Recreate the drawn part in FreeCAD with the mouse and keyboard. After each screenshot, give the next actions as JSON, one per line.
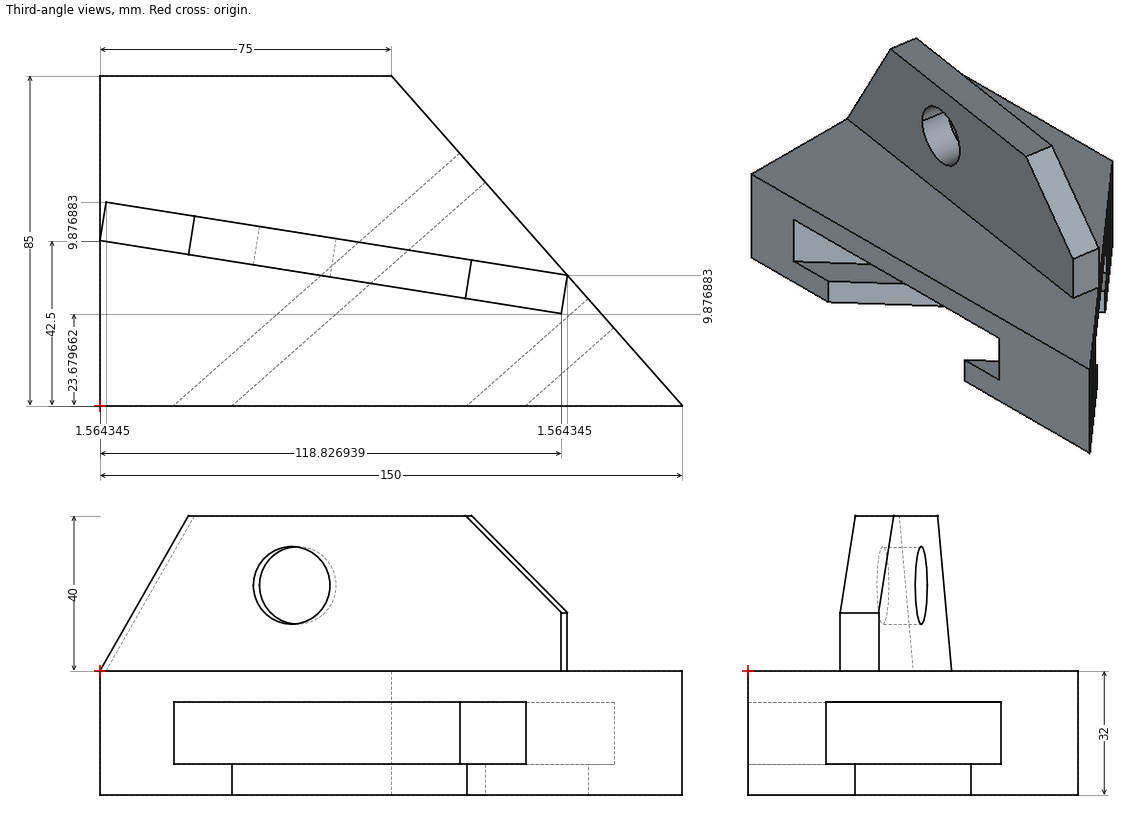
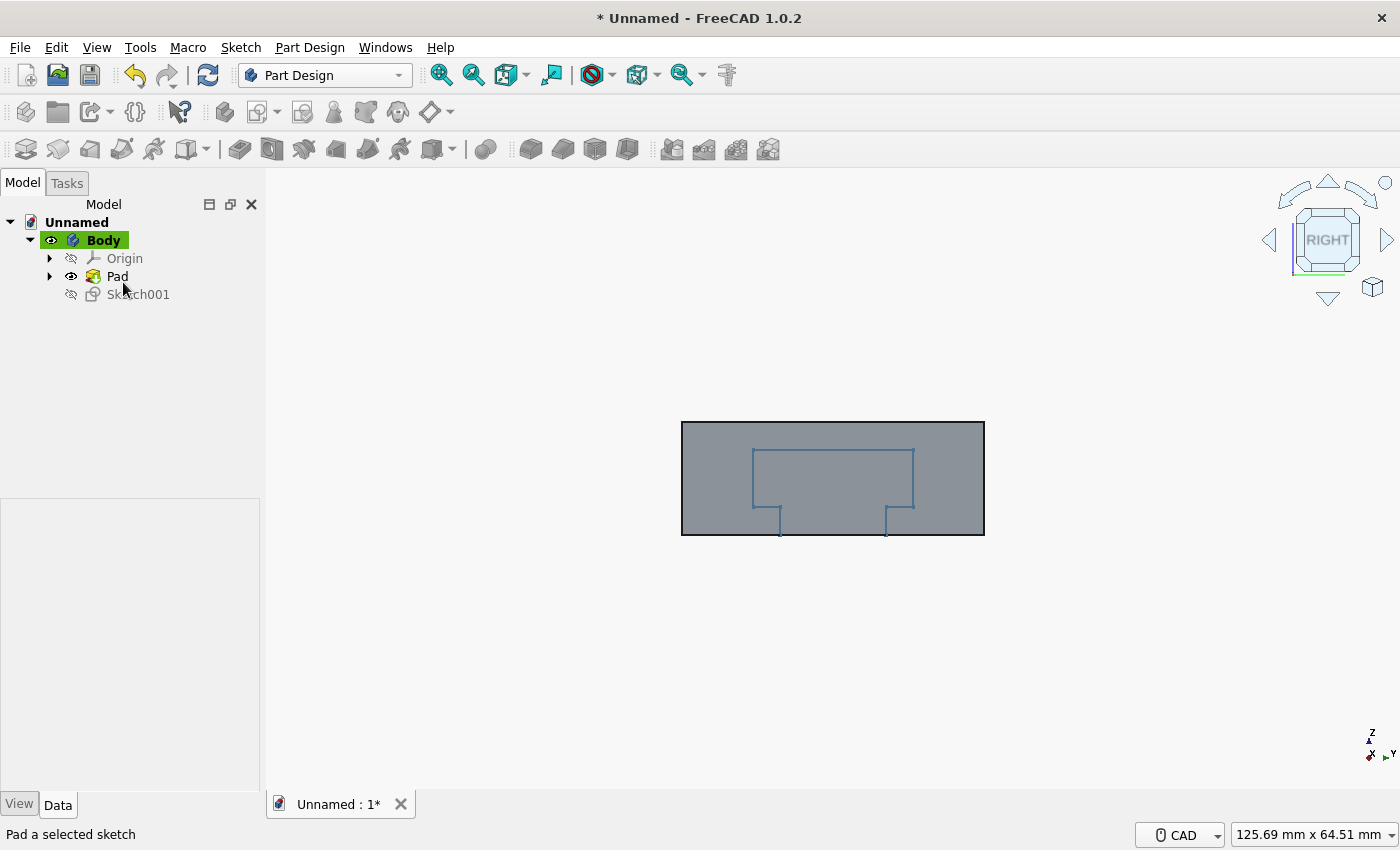
{"action": "left_click", "coordinate": [240, 150]}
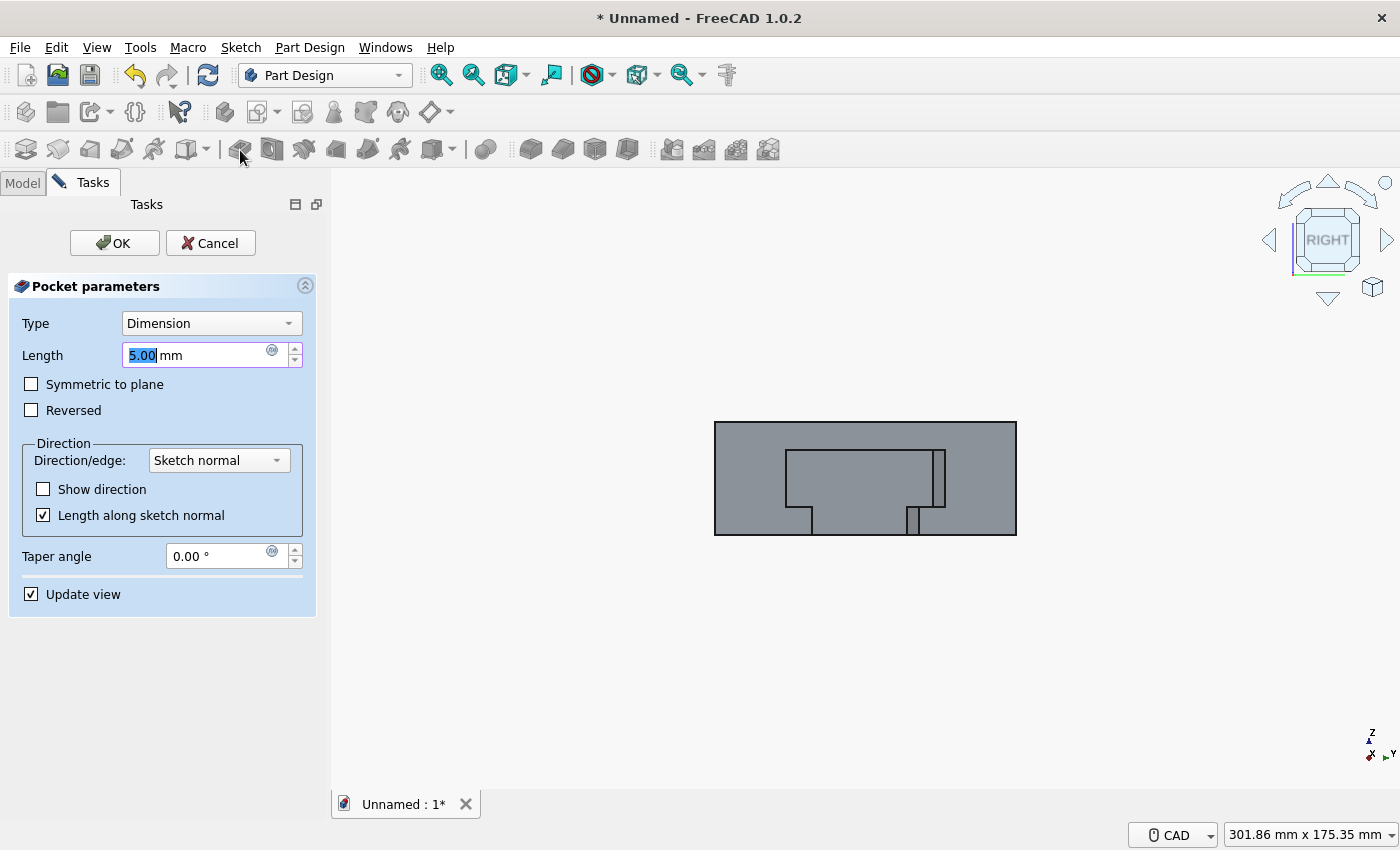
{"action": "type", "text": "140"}
{"action": "key", "text": "Tab"}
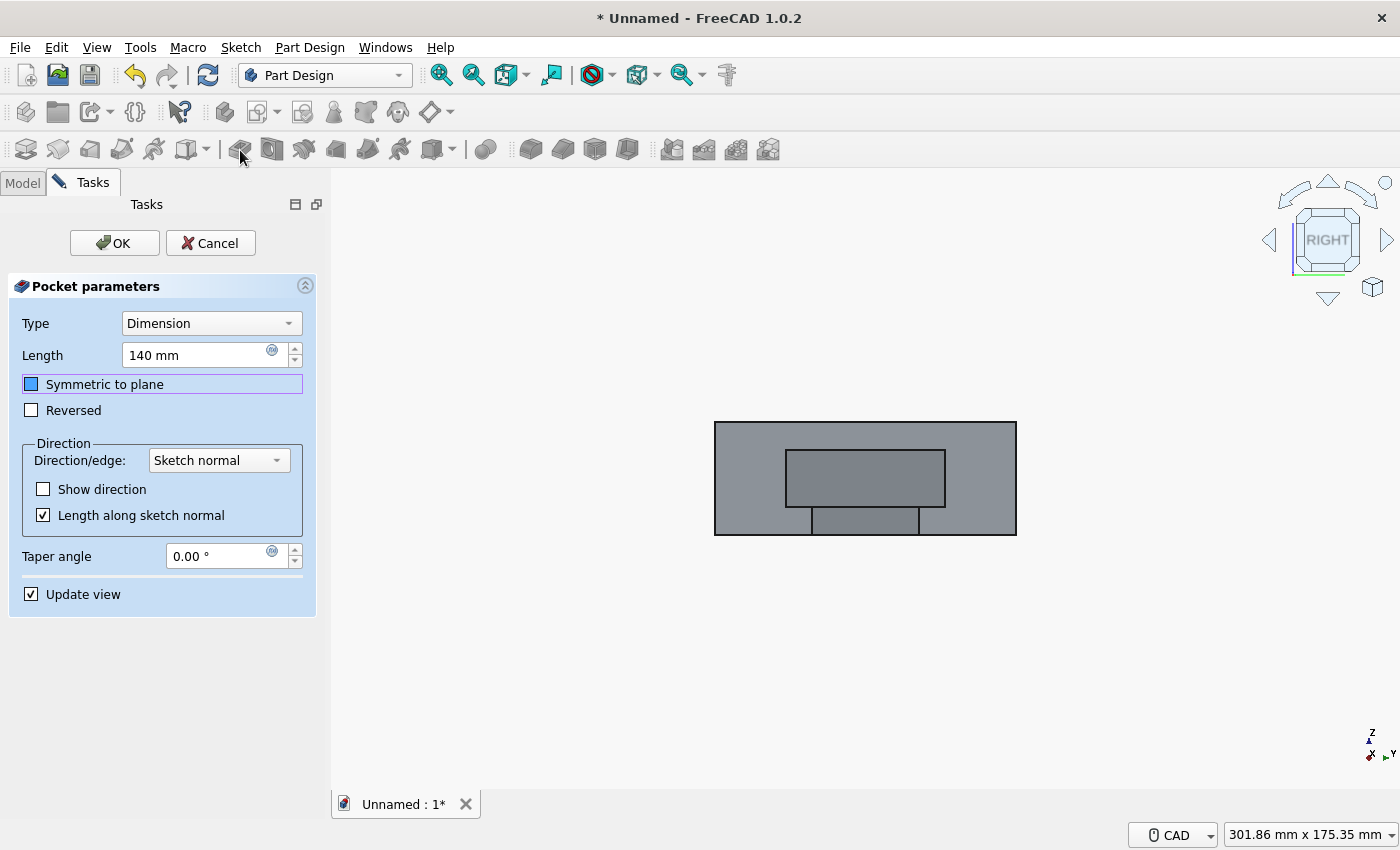
{"action": "left_click", "coordinate": [115, 243]}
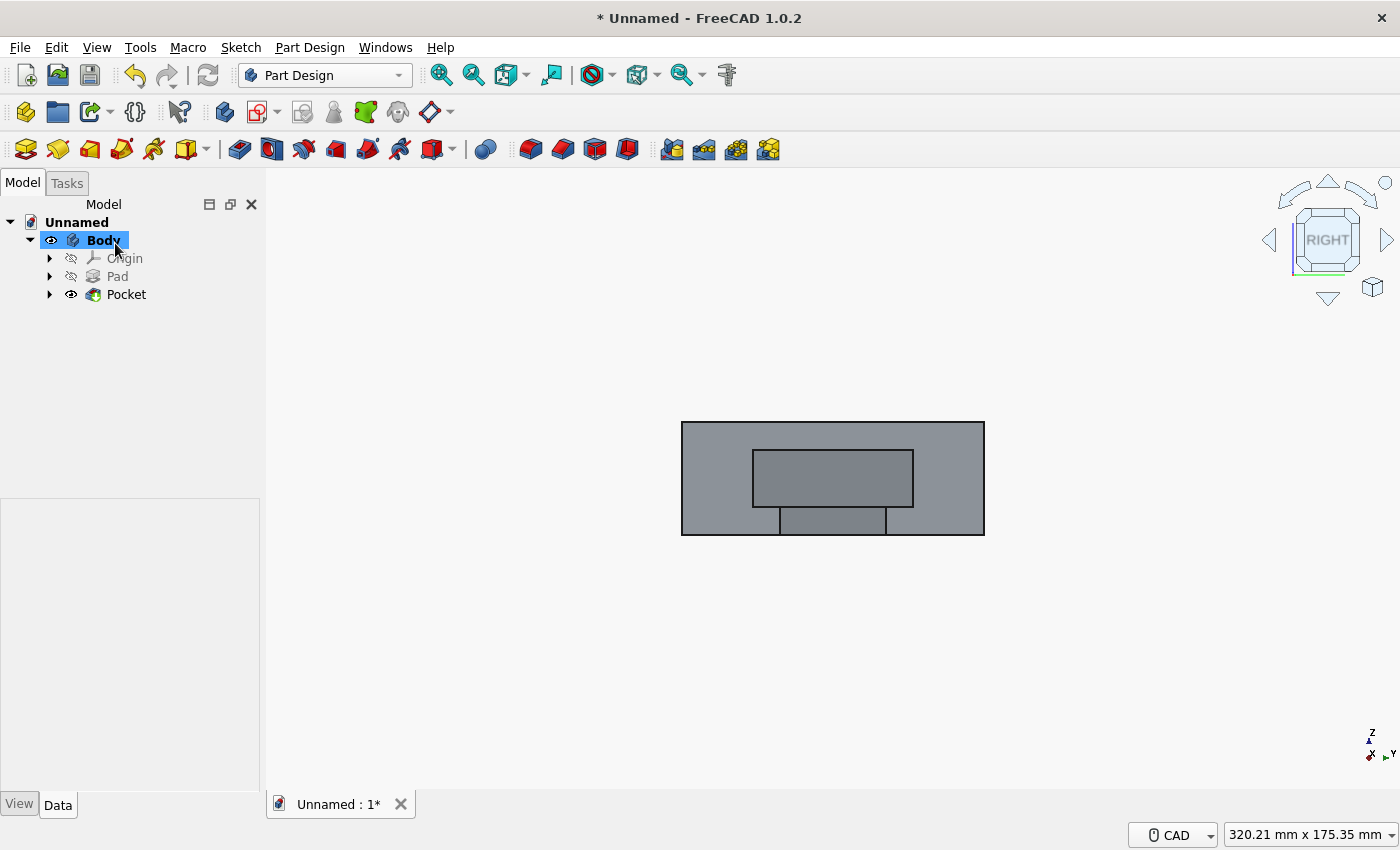
{"action": "key", "text": "v f"}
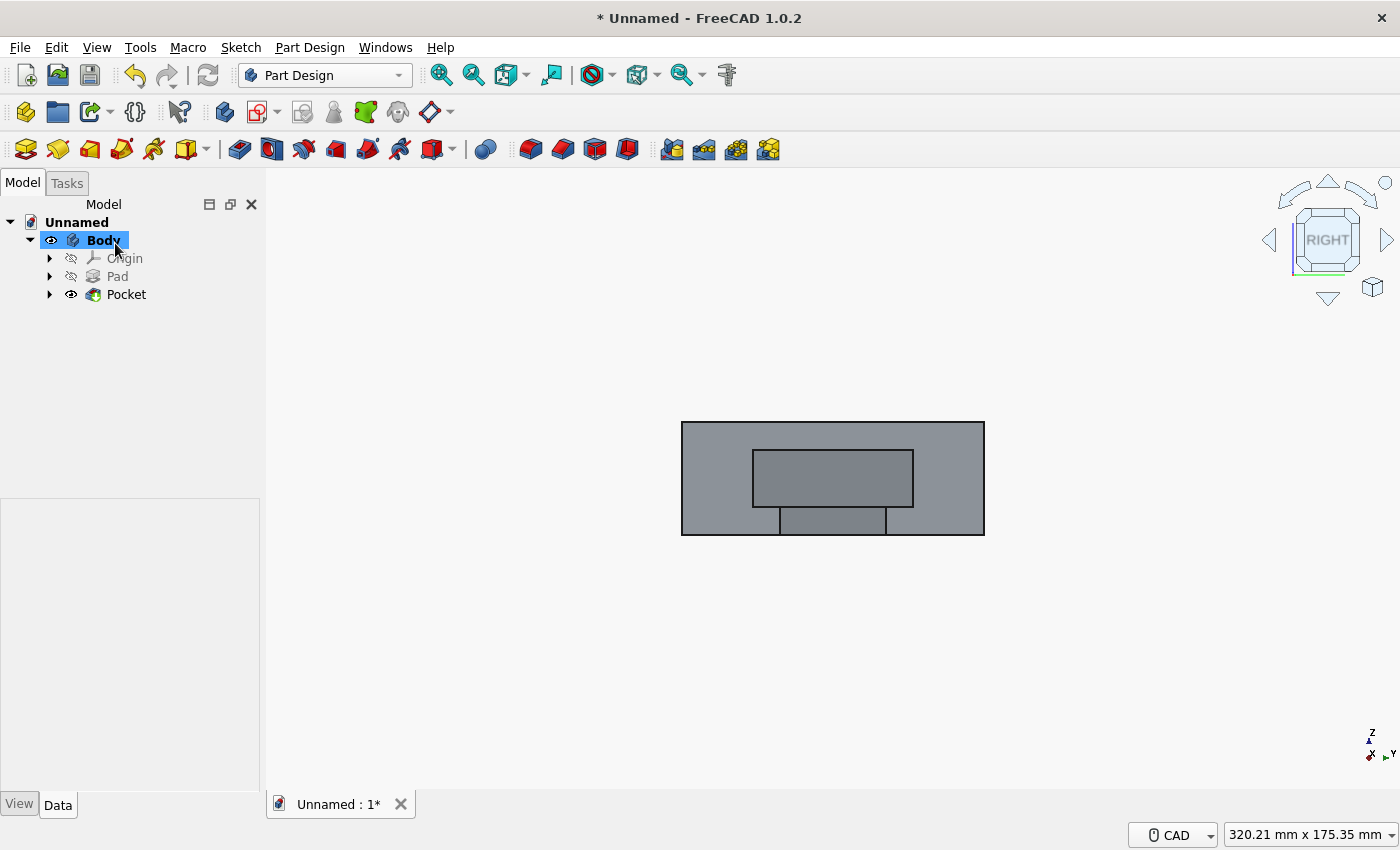
{"action": "key", "text": "0"}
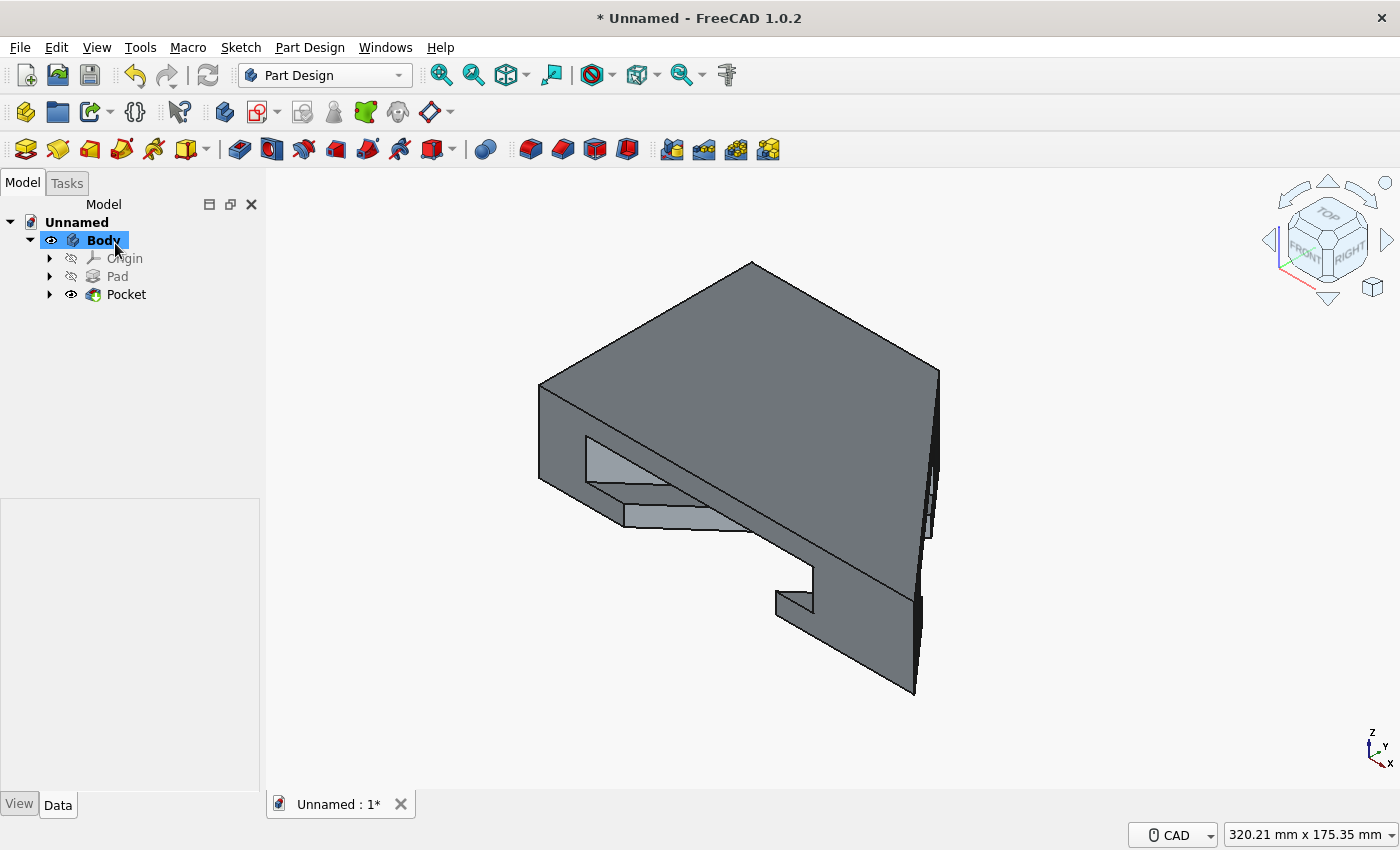
{"action": "left_click", "coordinate": [779, 400]}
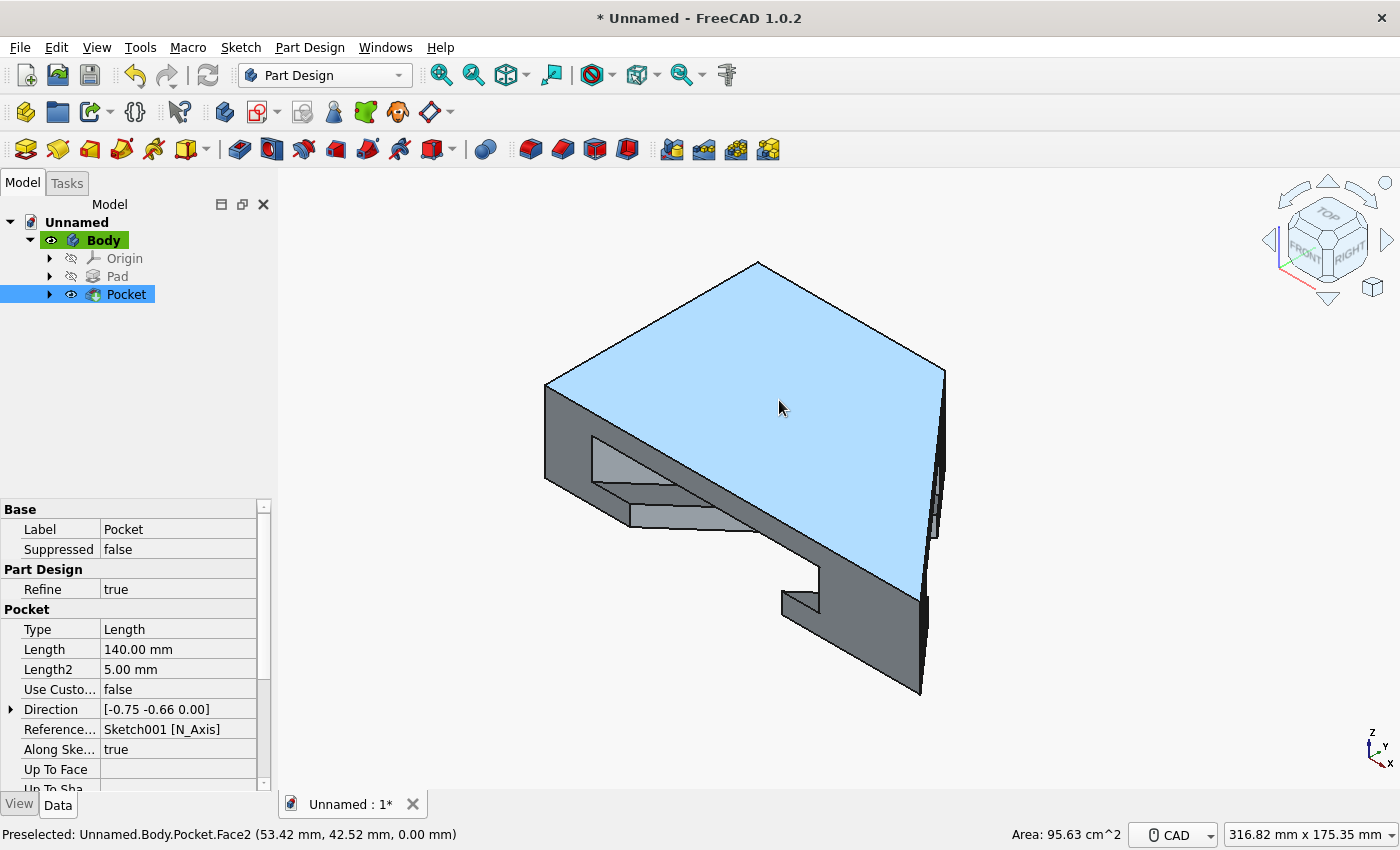
{"action": "left_click", "coordinate": [258, 112]}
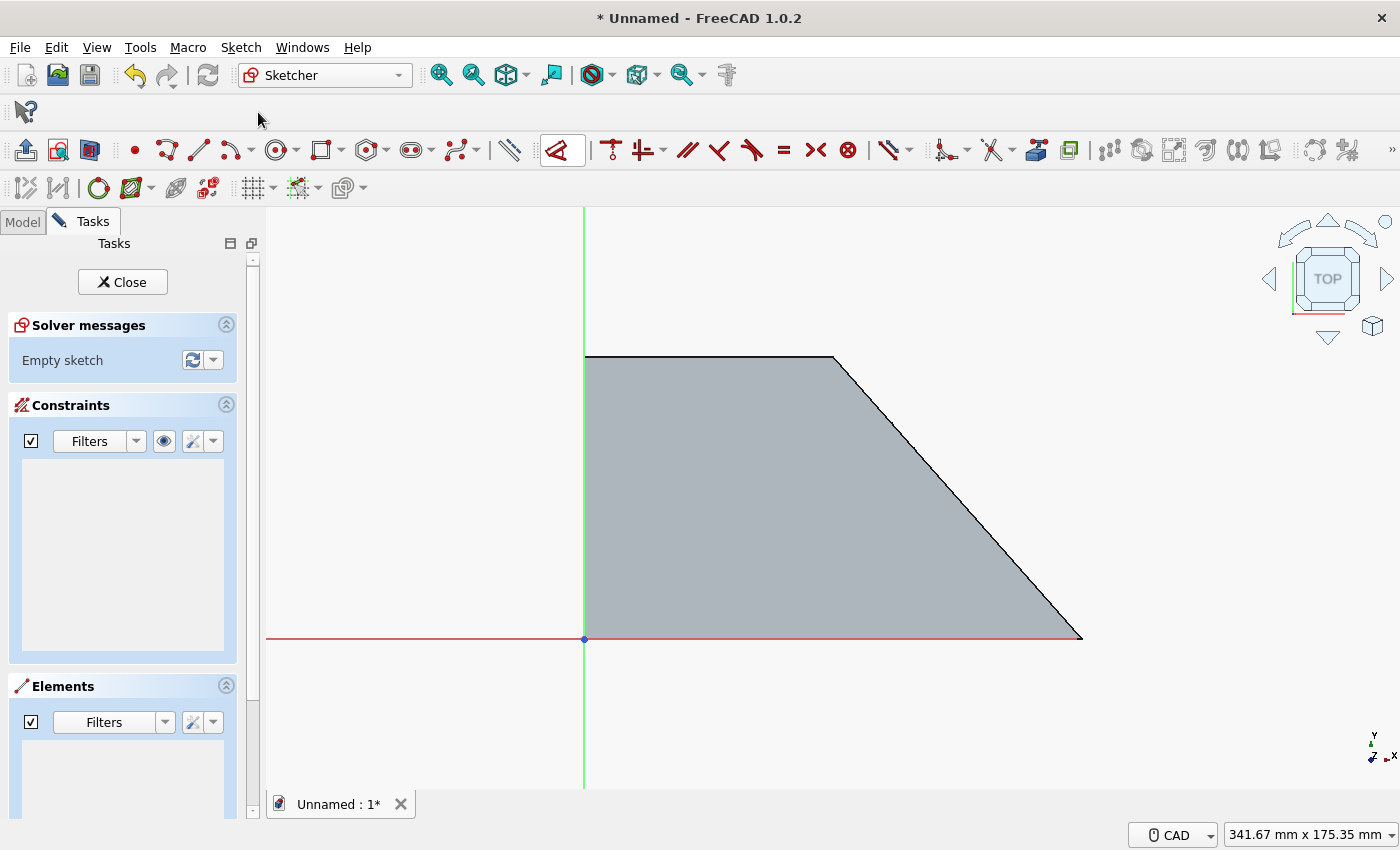
{"action": "scroll", "coordinate": [807, 618], "scroll_direction": "up", "scroll_amount": 3}